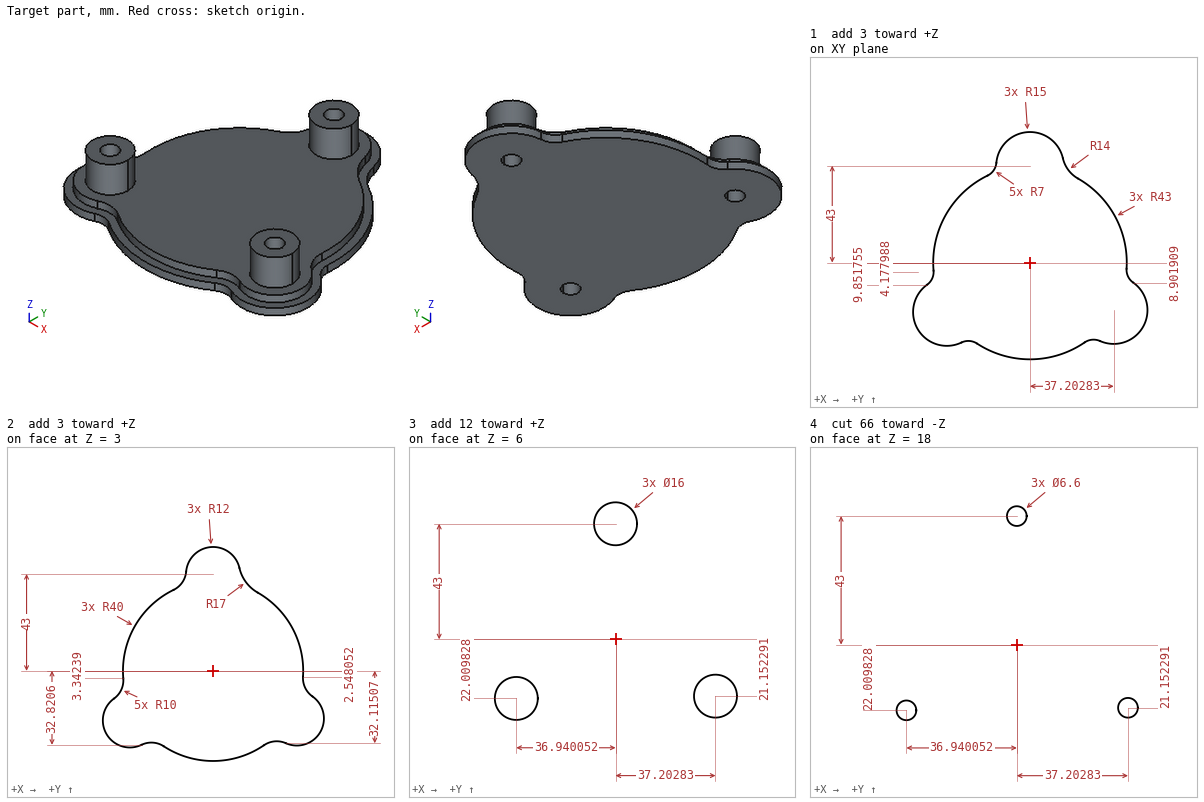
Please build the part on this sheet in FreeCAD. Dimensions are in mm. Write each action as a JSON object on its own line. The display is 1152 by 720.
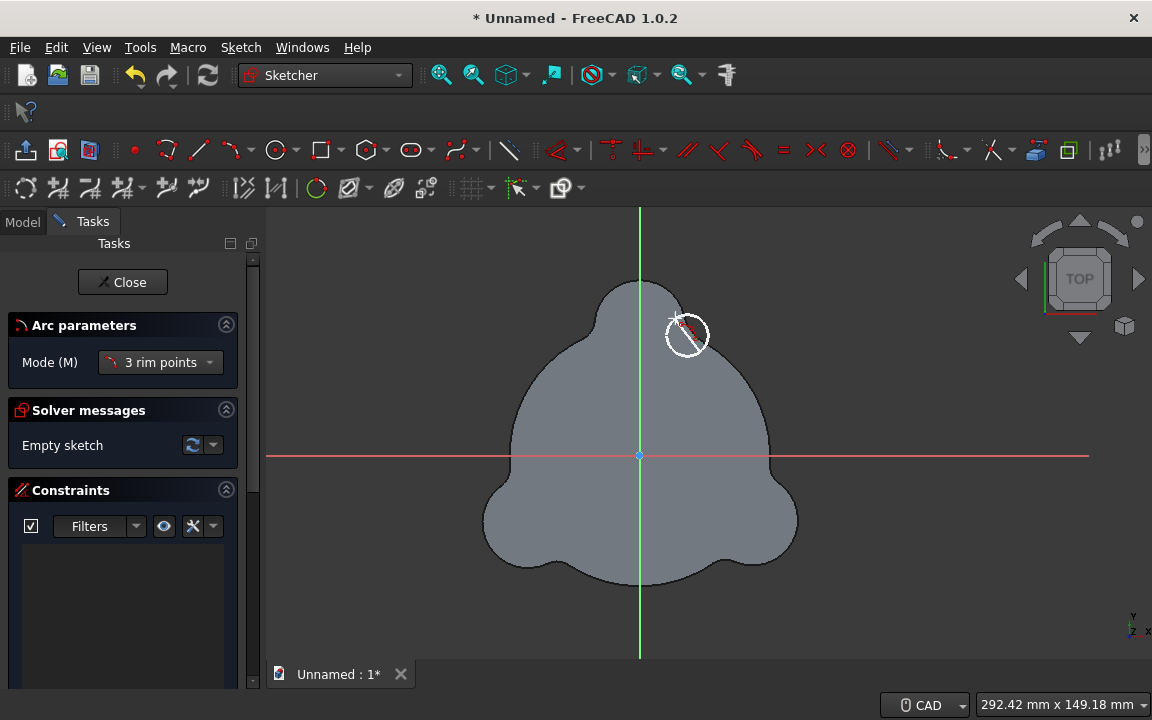
{"action": "scroll", "coordinate": [684, 337], "scroll_direction": "up", "scroll_amount": 7}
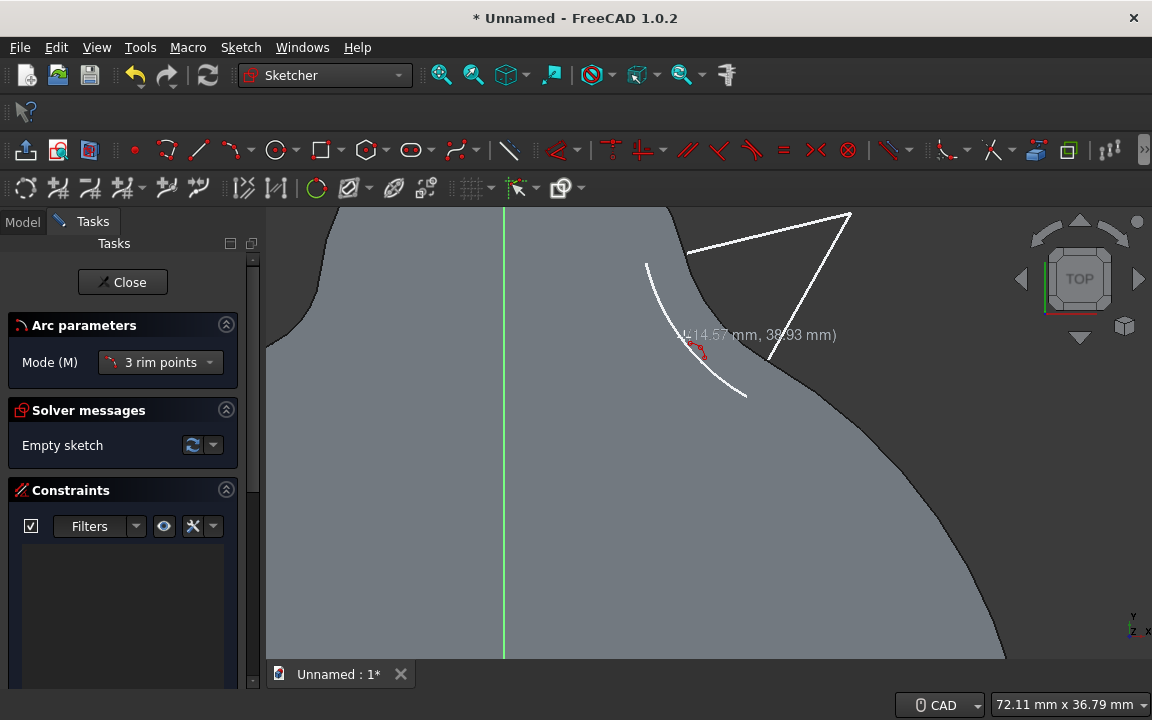
{"action": "left_click", "coordinate": [683, 335]}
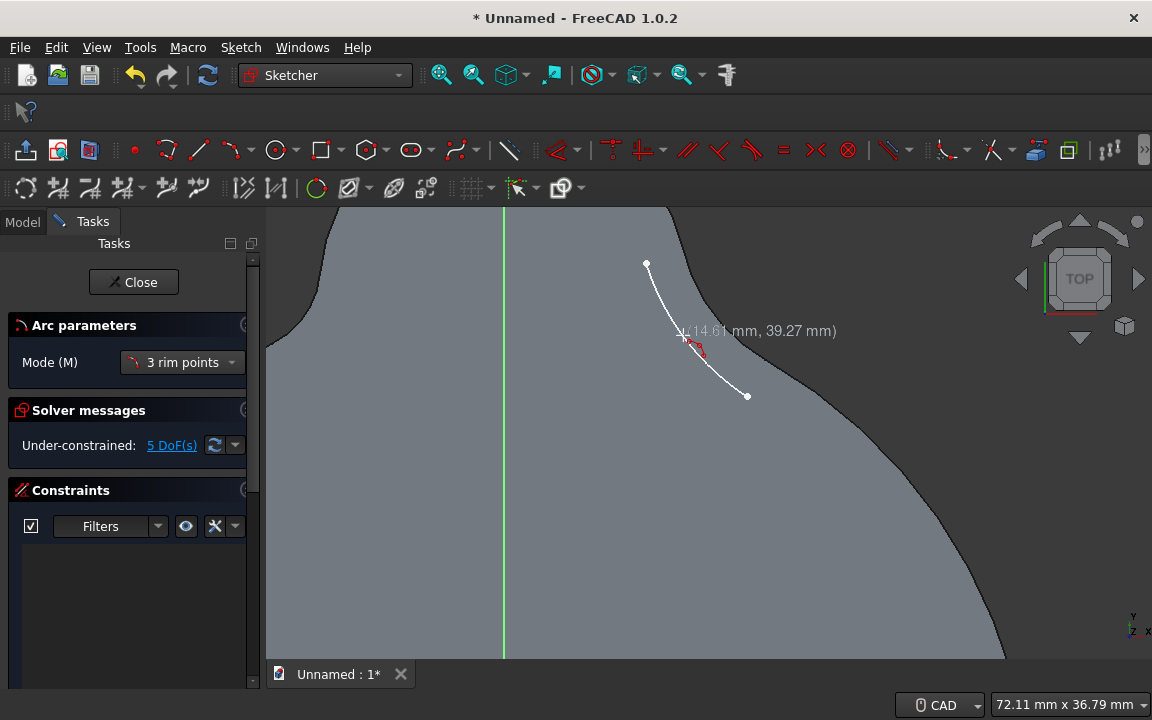
{"action": "scroll", "coordinate": [685, 337], "scroll_direction": "down", "scroll_amount": 7}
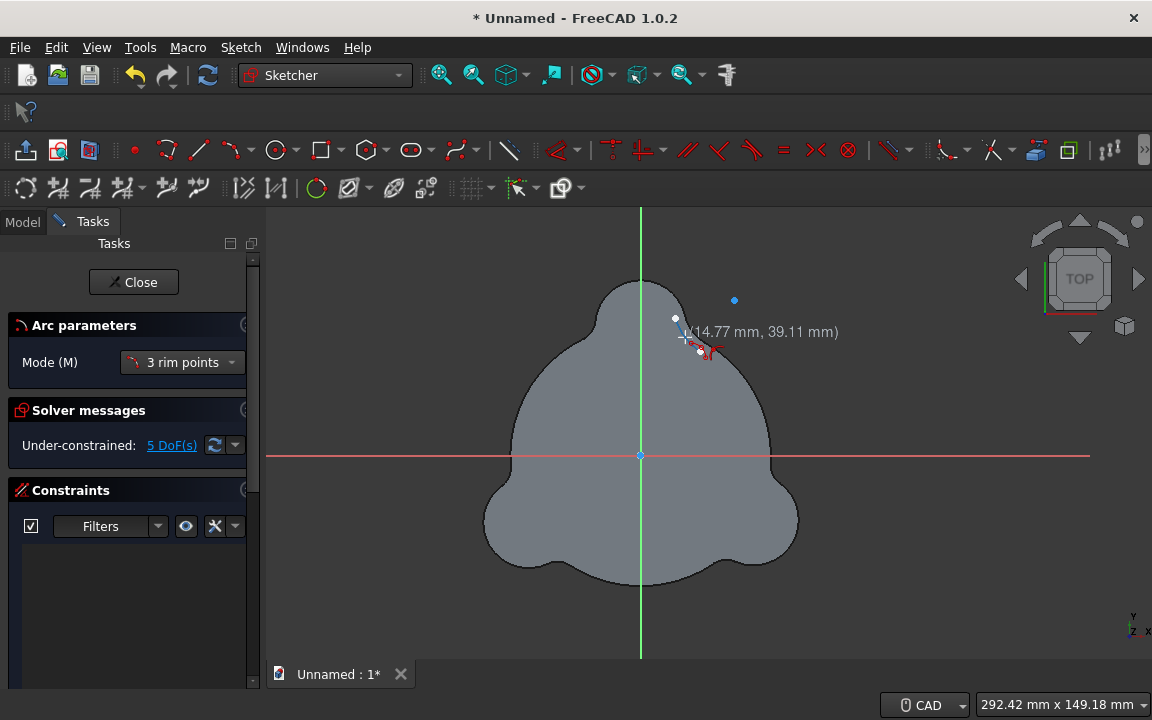
{"action": "left_click", "coordinate": [676, 319]}
{"action": "left_click", "coordinate": [604, 322]}
{"action": "left_click", "coordinate": [658, 294]}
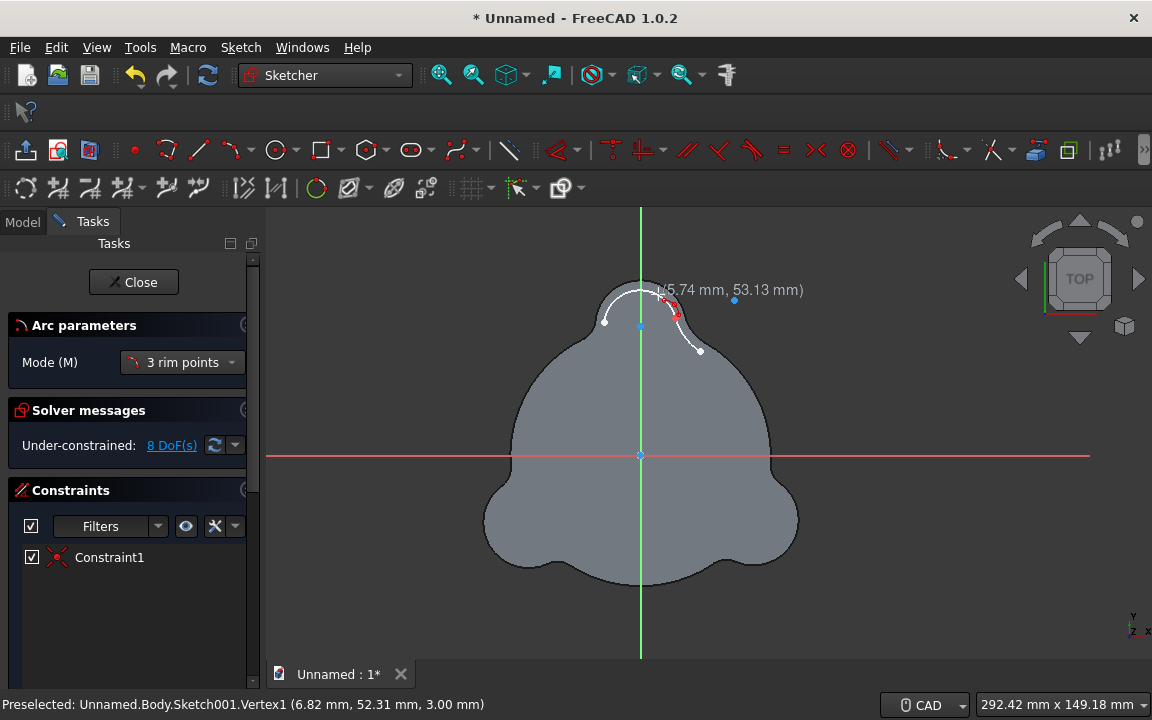
{"action": "left_click", "coordinate": [604, 323]}
{"action": "left_click", "coordinate": [587, 347]}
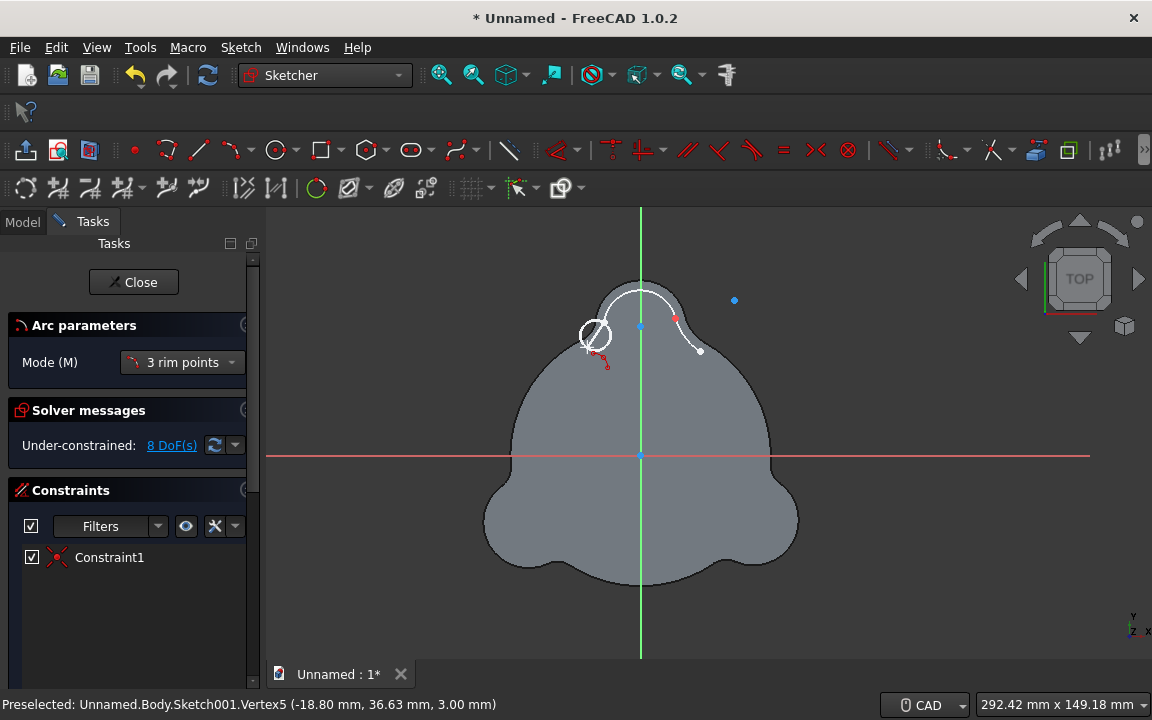
{"action": "scroll", "coordinate": [599, 337], "scroll_direction": "up", "scroll_amount": 7}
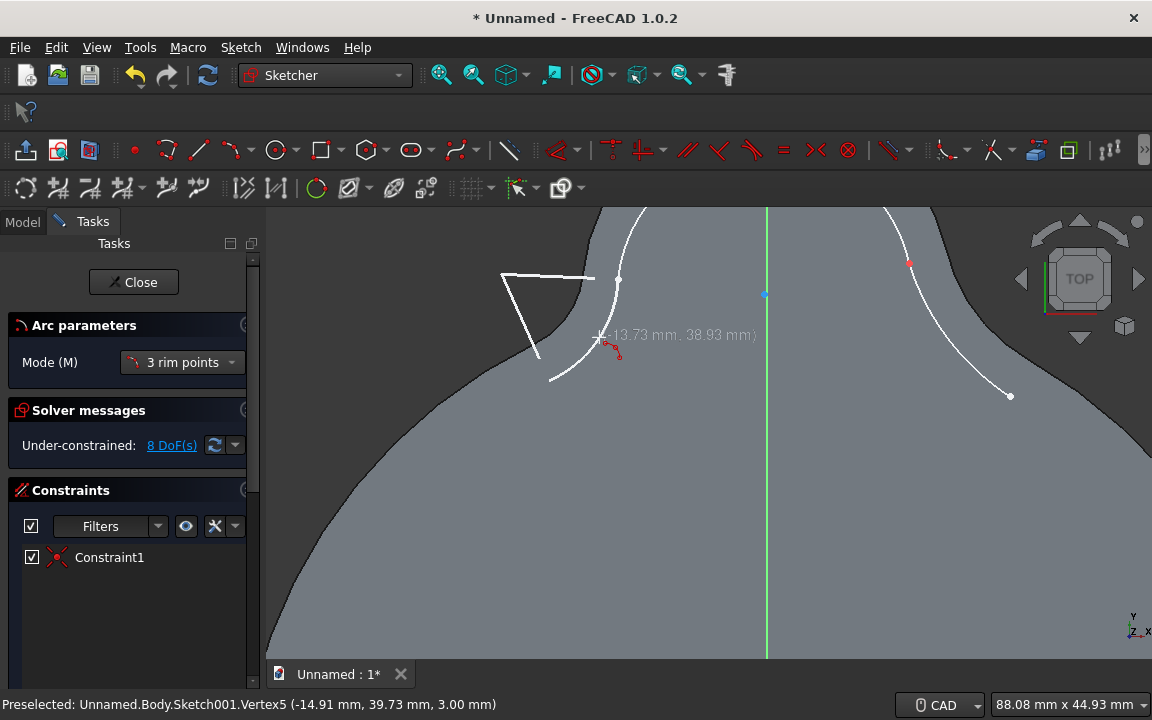
{"action": "left_click", "coordinate": [599, 336]}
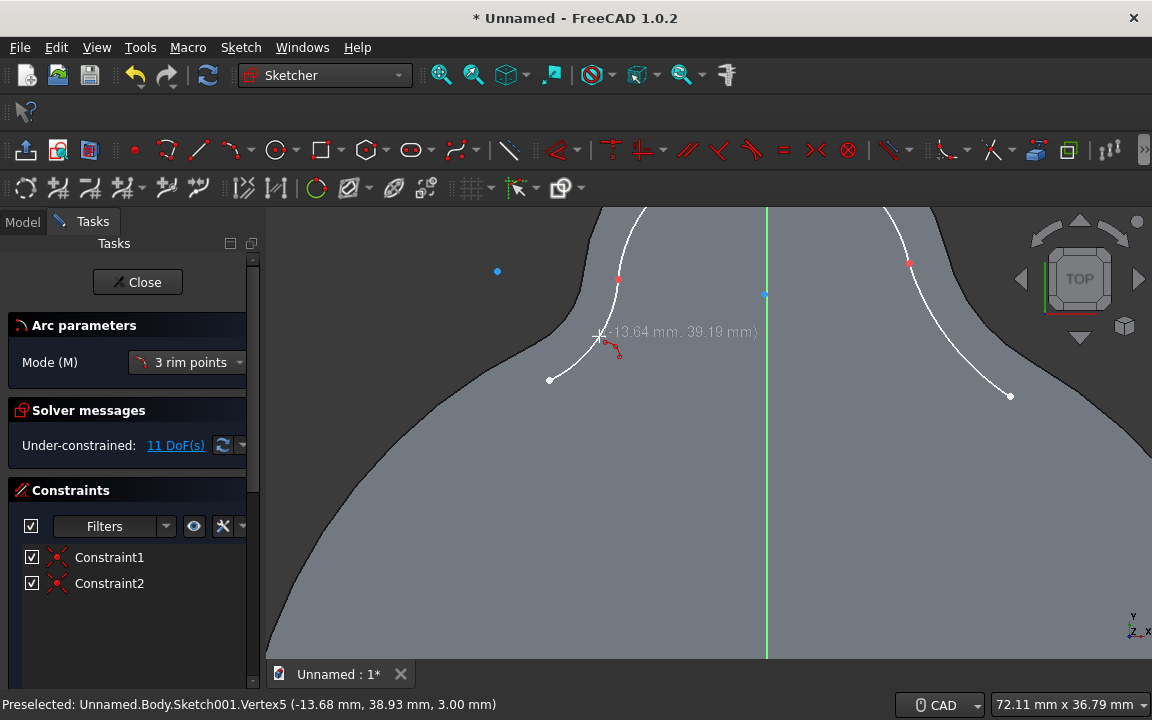
{"action": "scroll", "coordinate": [598, 337], "scroll_direction": "down", "scroll_amount": 7}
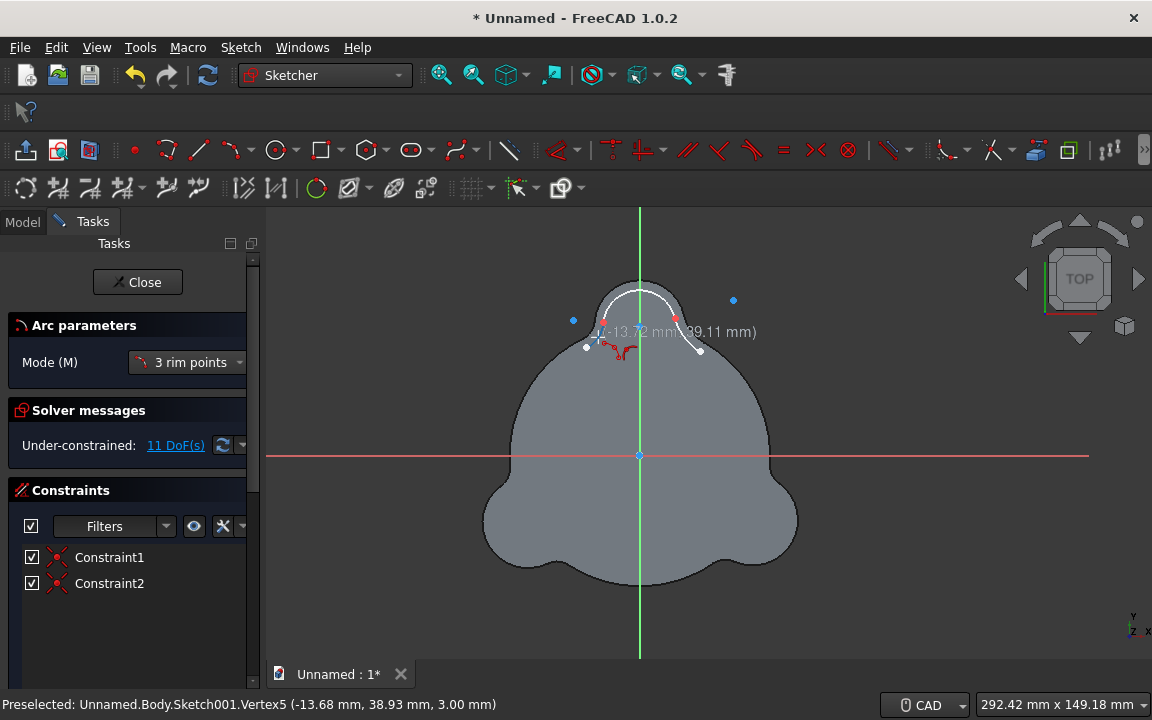
{"action": "left_click", "coordinate": [586, 348]}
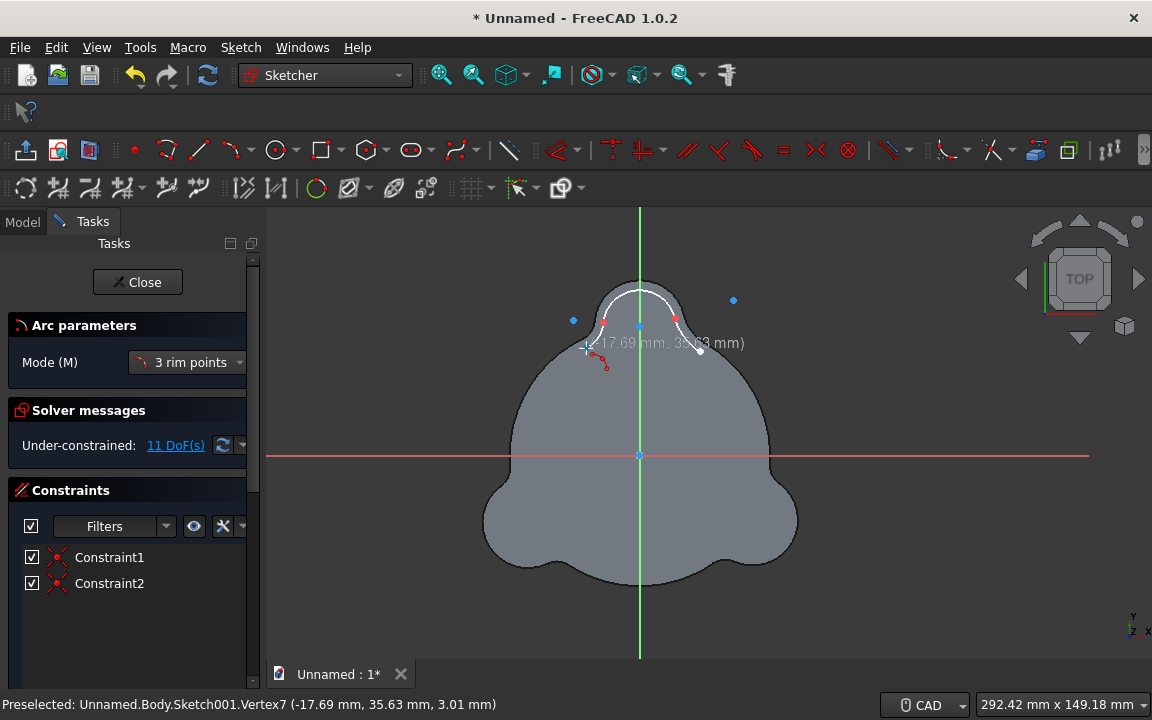
{"action": "scroll", "coordinate": [519, 466], "scroll_direction": "up", "scroll_amount": 3}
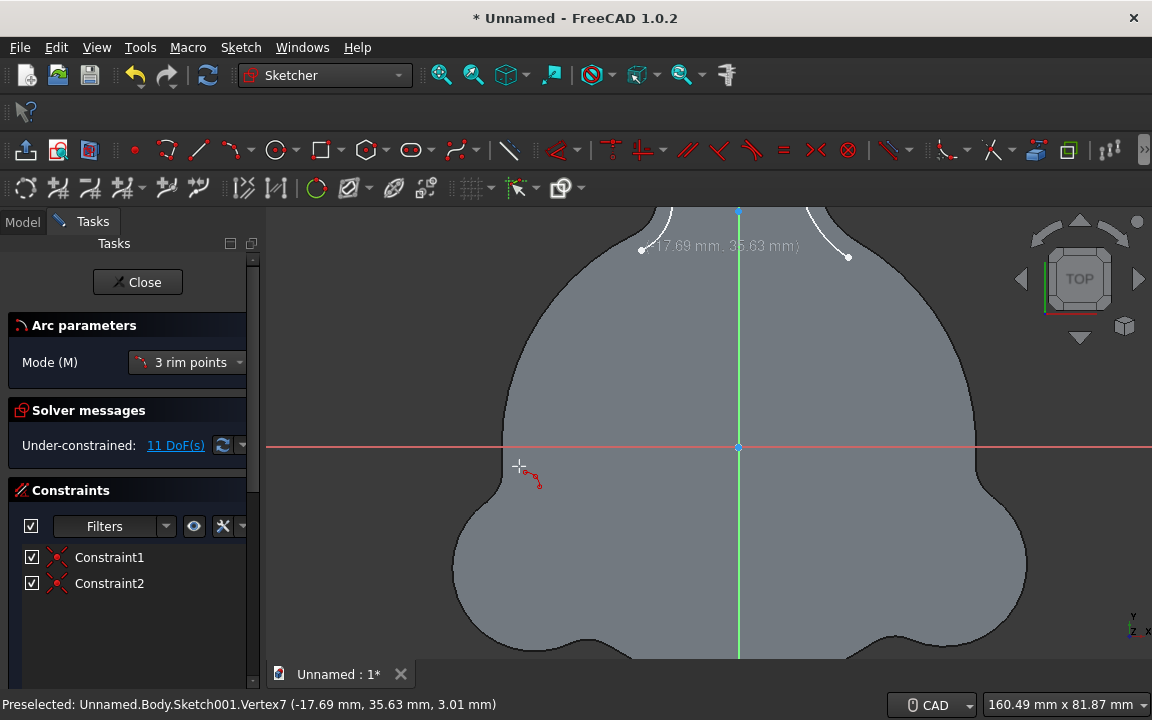
{"action": "left_click", "coordinate": [519, 466]}
{"action": "left_click", "coordinate": [547, 338]}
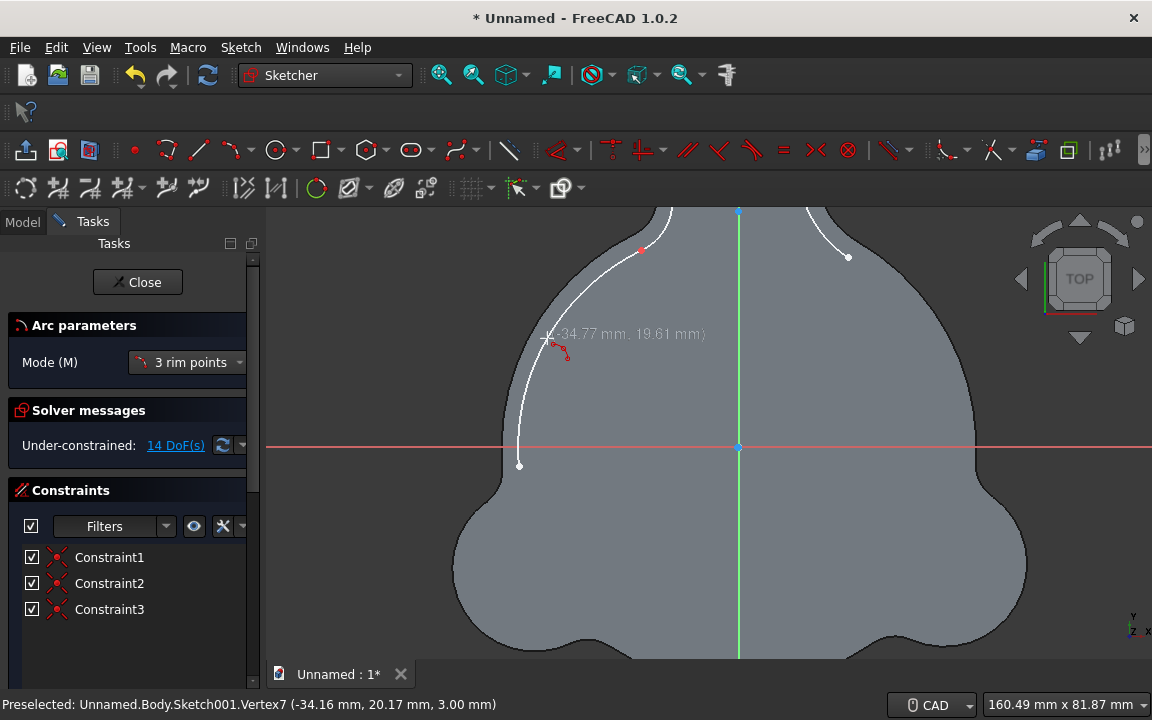
{"action": "left_click", "coordinate": [519, 467]}
{"action": "left_click", "coordinate": [496, 515]}